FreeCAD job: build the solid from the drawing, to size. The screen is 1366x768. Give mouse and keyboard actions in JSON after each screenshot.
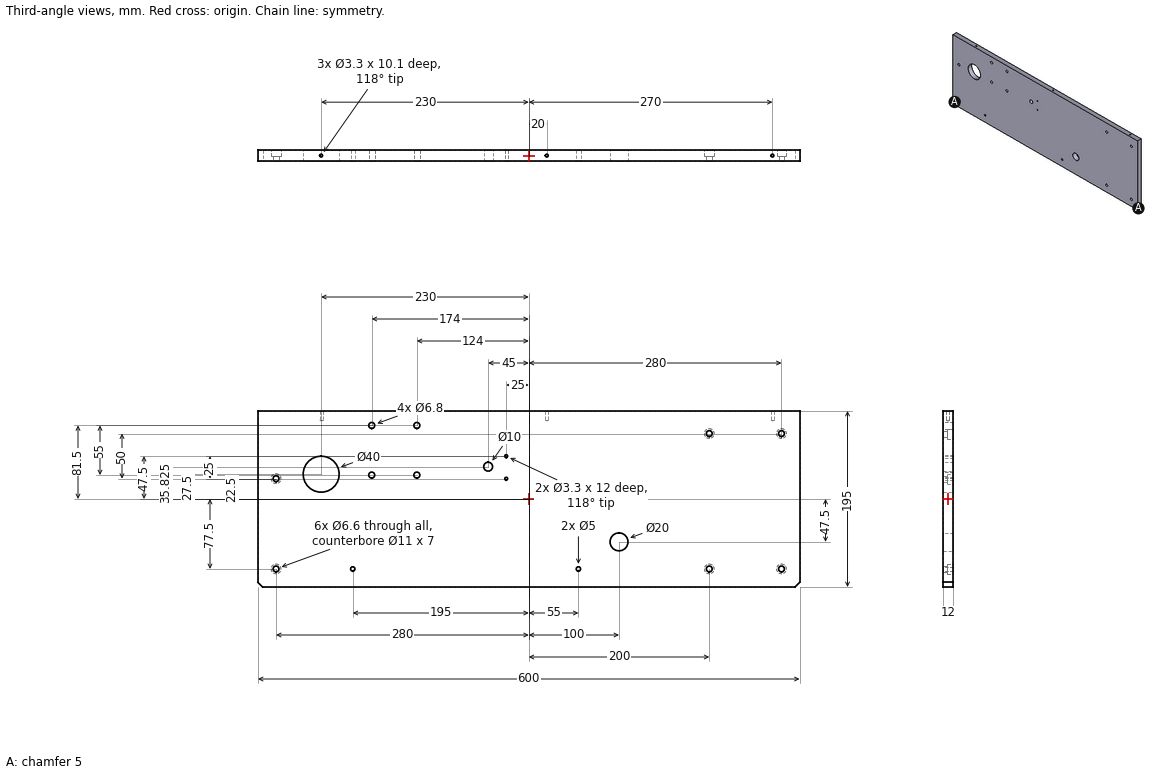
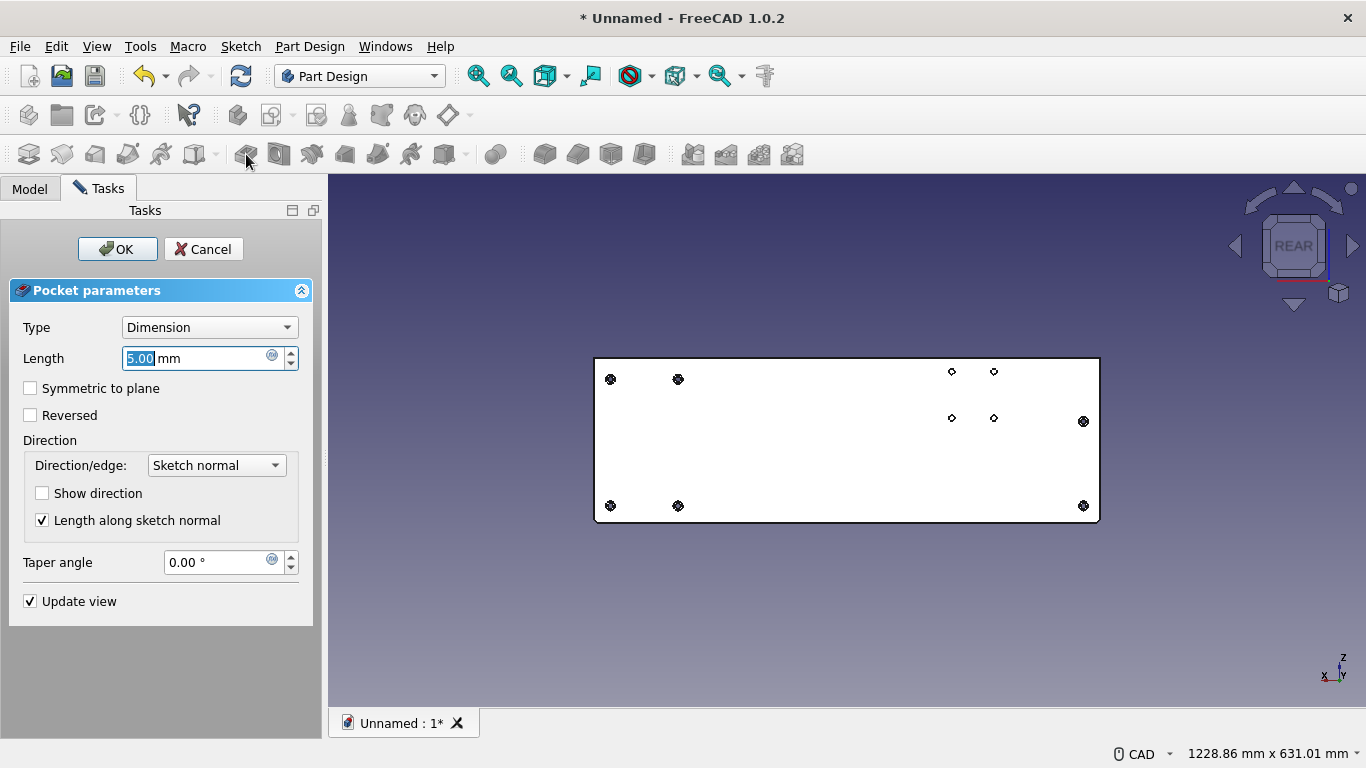
{"action": "left_click", "coordinate": [210, 328]}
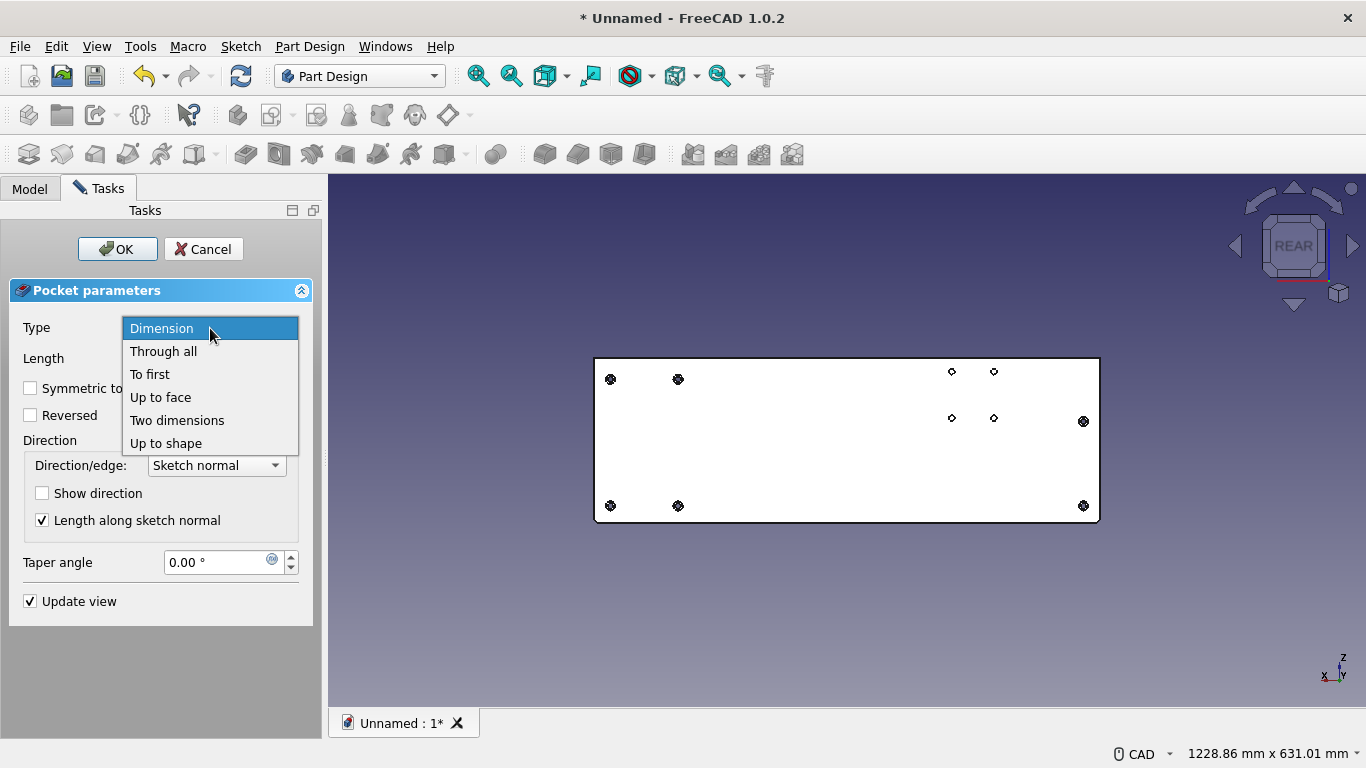
{"action": "left_click", "coordinate": [208, 352]}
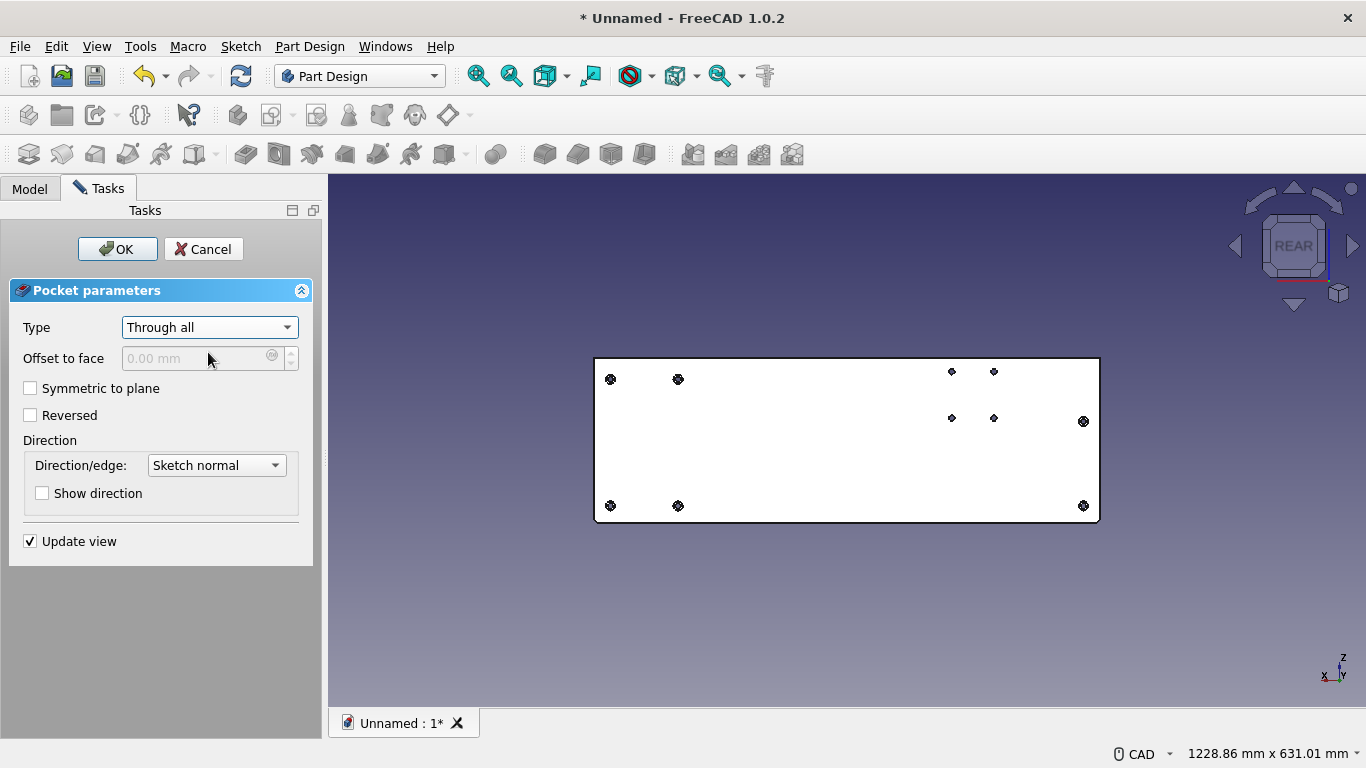
{"action": "left_click", "coordinate": [118, 249]}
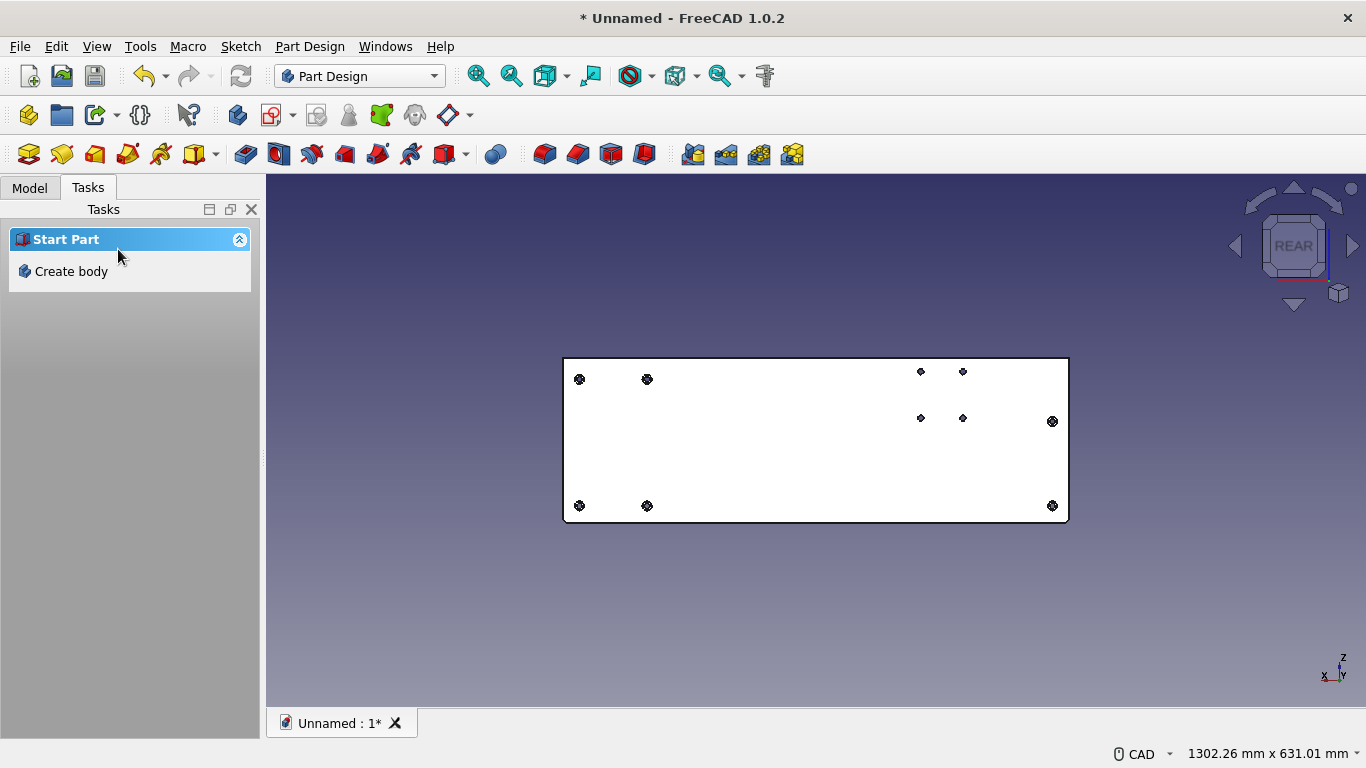
{"action": "left_click", "coordinate": [744, 439]}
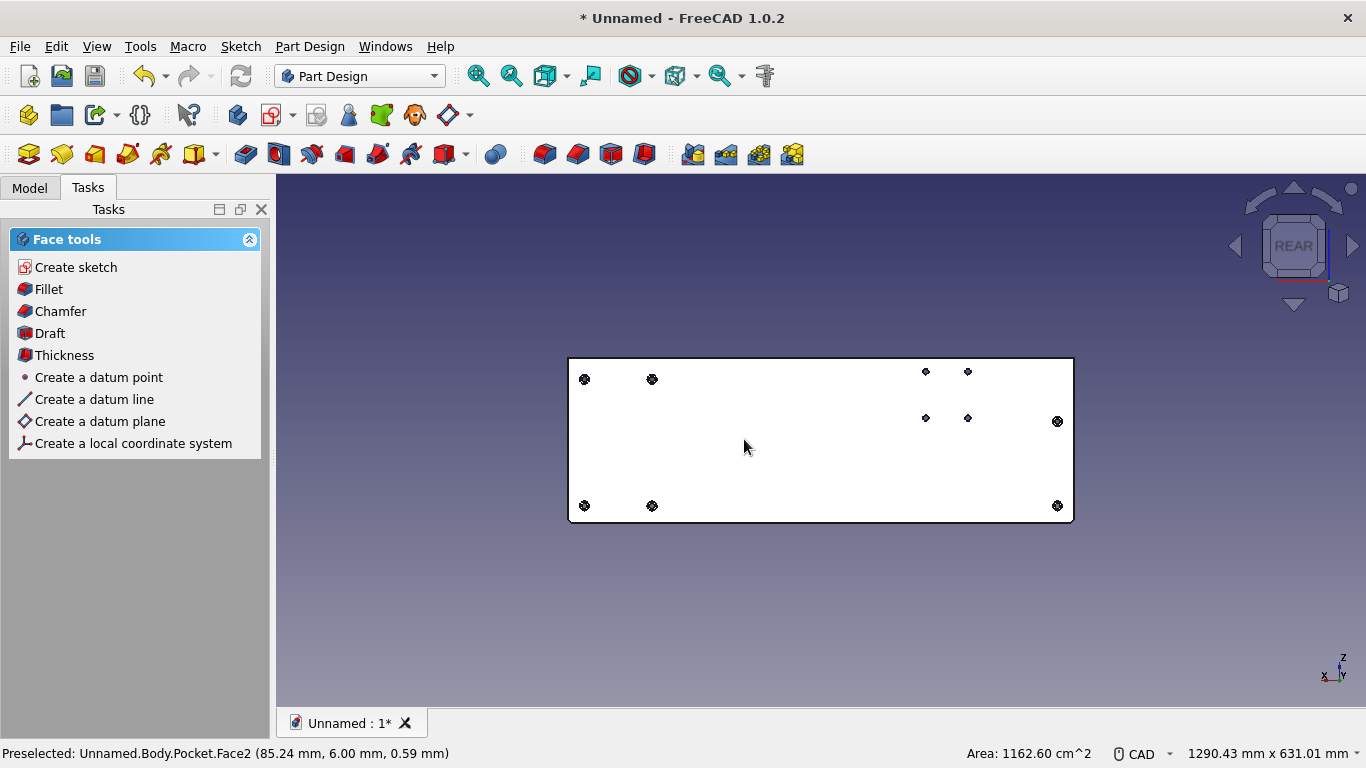
{"action": "left_click", "coordinate": [270, 116]}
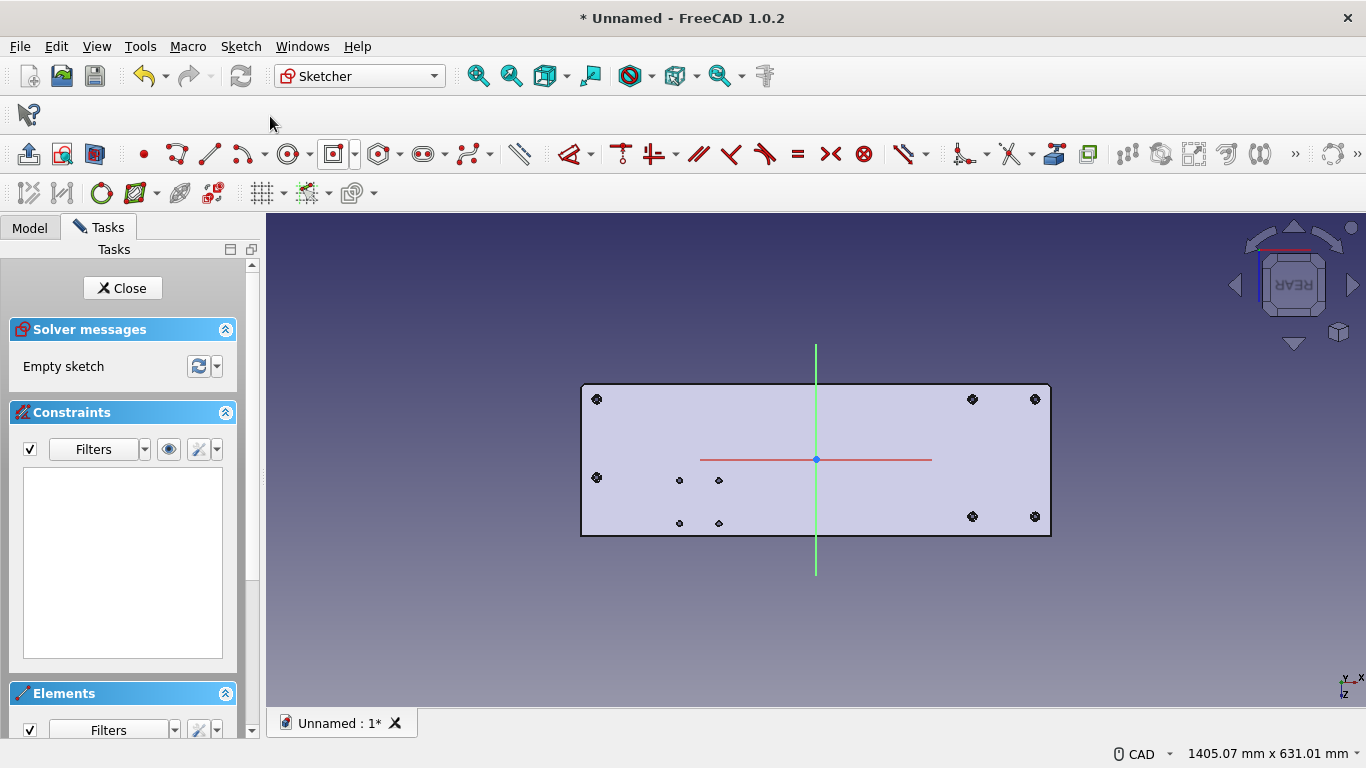
{"action": "scroll", "coordinate": [767, 415], "scroll_direction": "up", "scroll_amount": 6}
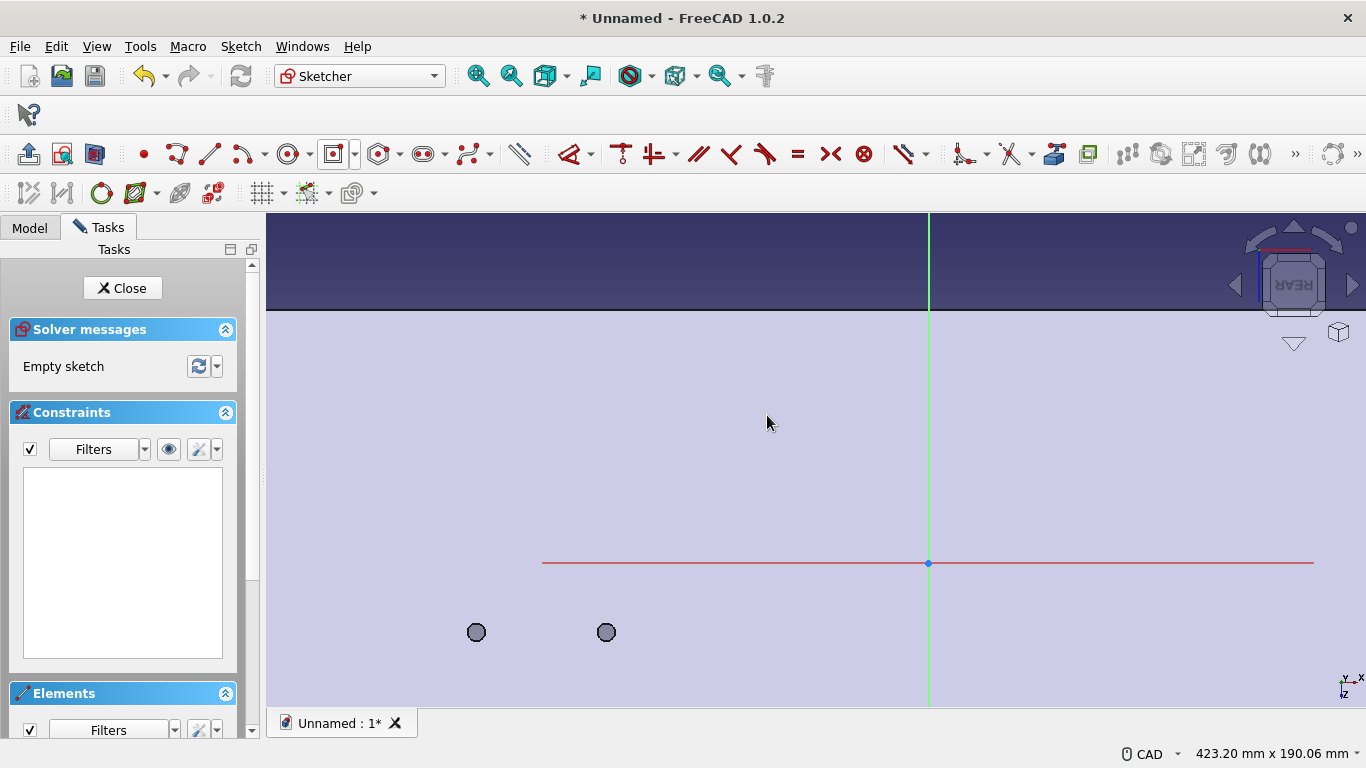
{"action": "left_click", "coordinate": [288, 154]}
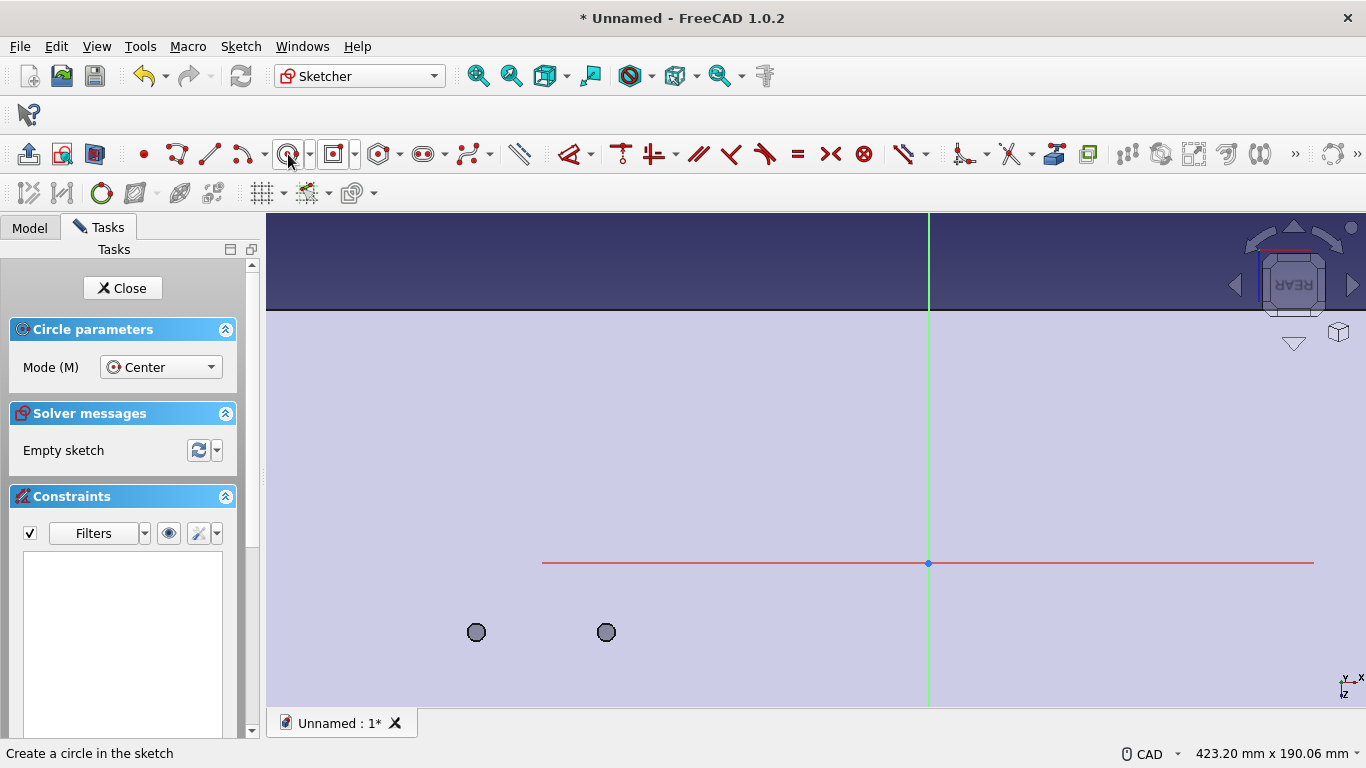
{"action": "scroll", "coordinate": [1072, 362], "scroll_direction": "up", "scroll_amount": 7}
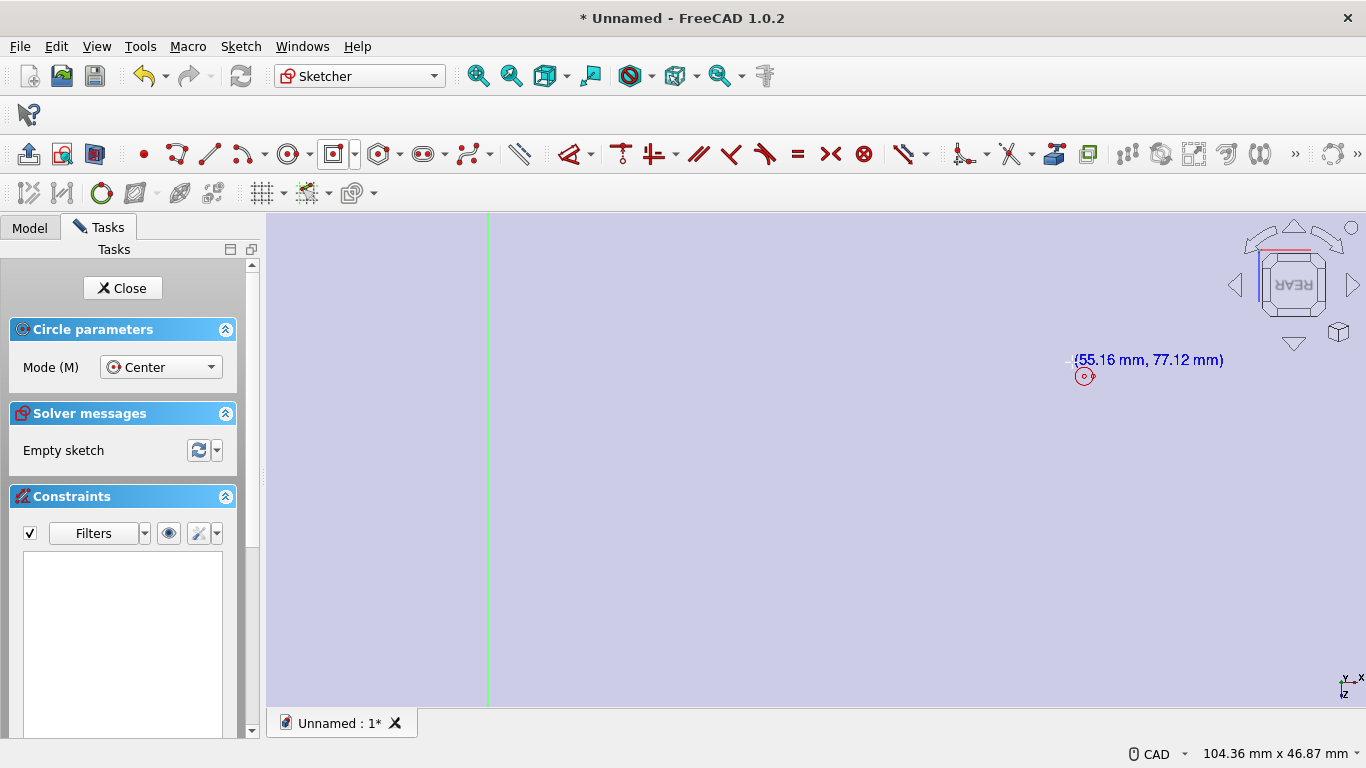
{"action": "scroll", "coordinate": [1074, 363], "scroll_direction": "down", "scroll_amount": 7}